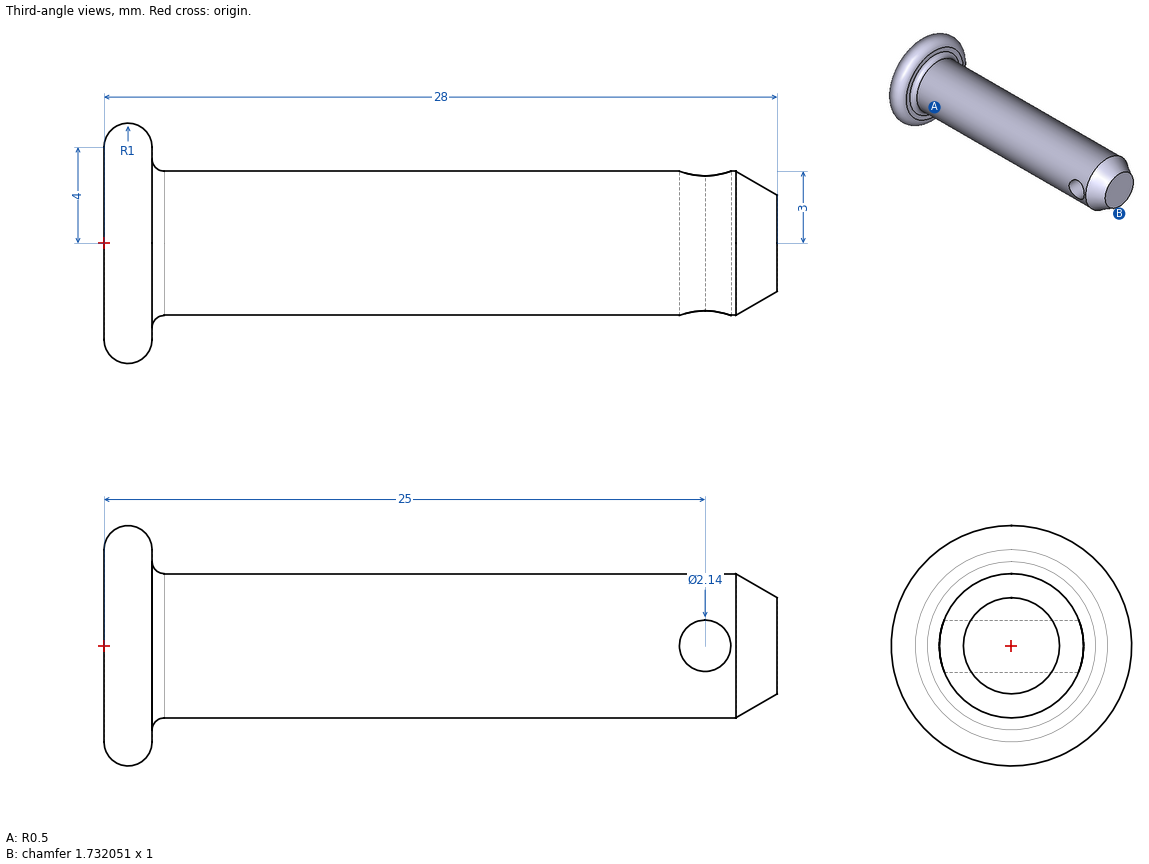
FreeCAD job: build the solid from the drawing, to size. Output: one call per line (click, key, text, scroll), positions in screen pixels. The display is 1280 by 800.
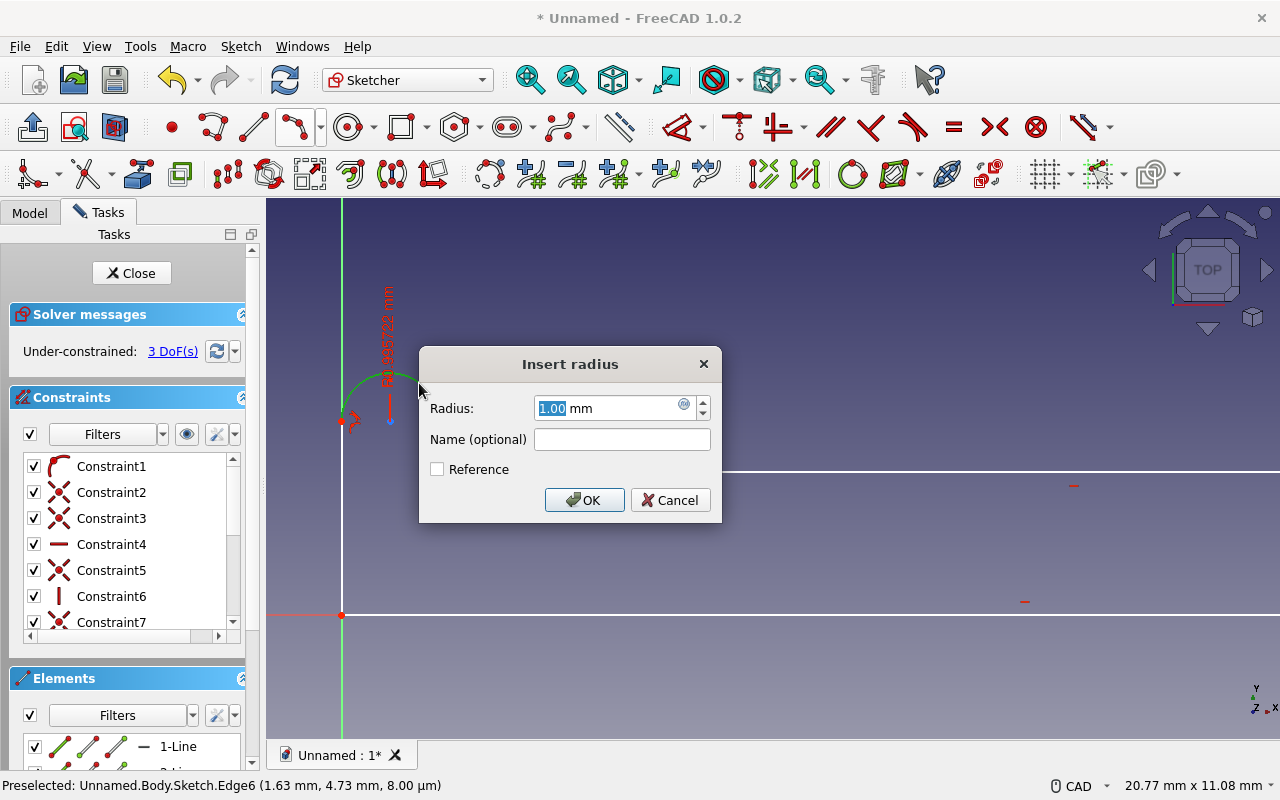
text(1)
key(Return)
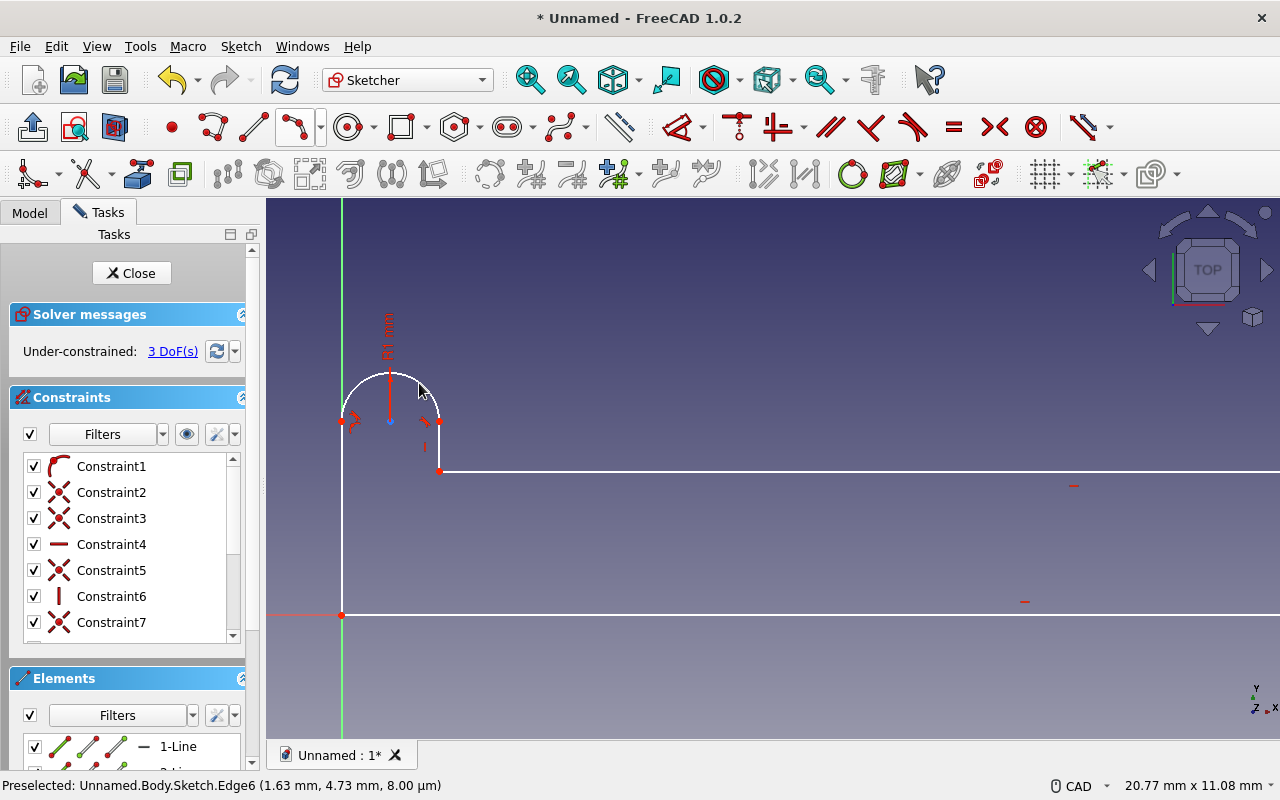
click(342, 480)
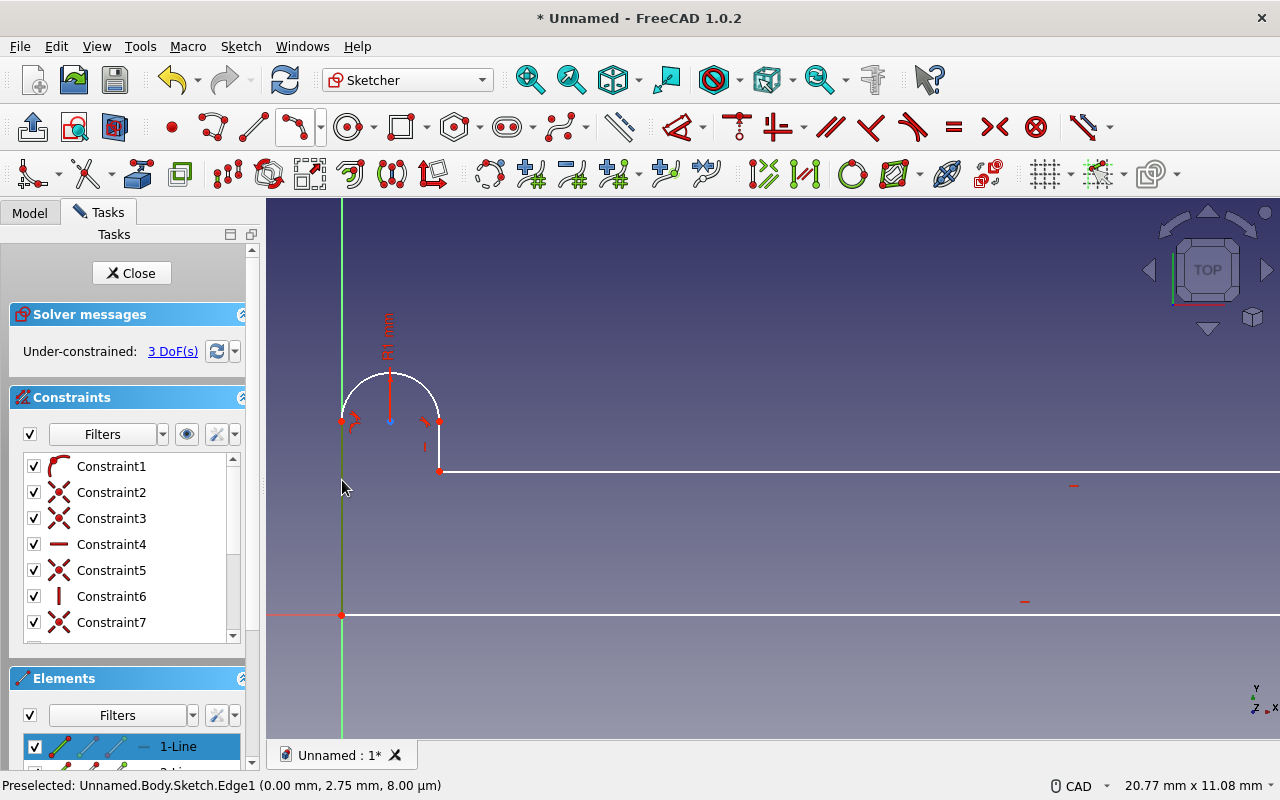
key(i)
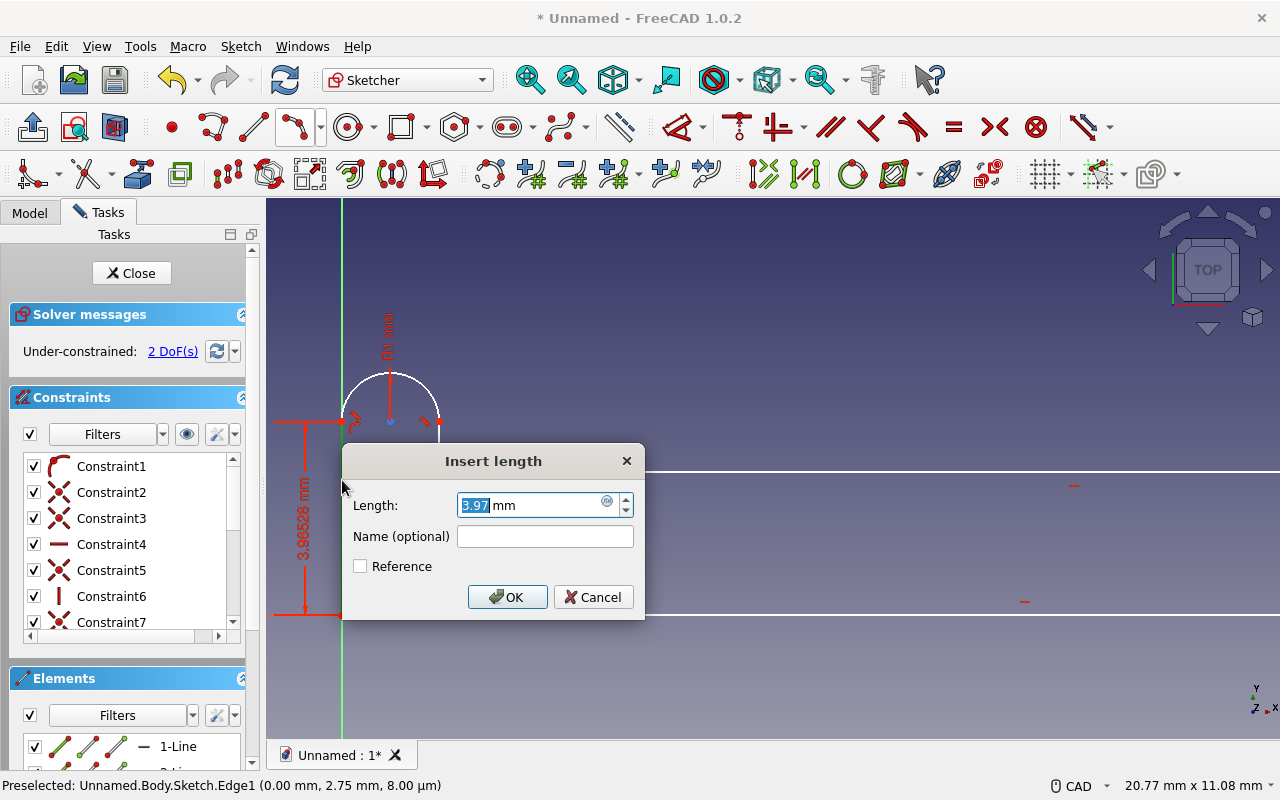
text(4)
key(Return)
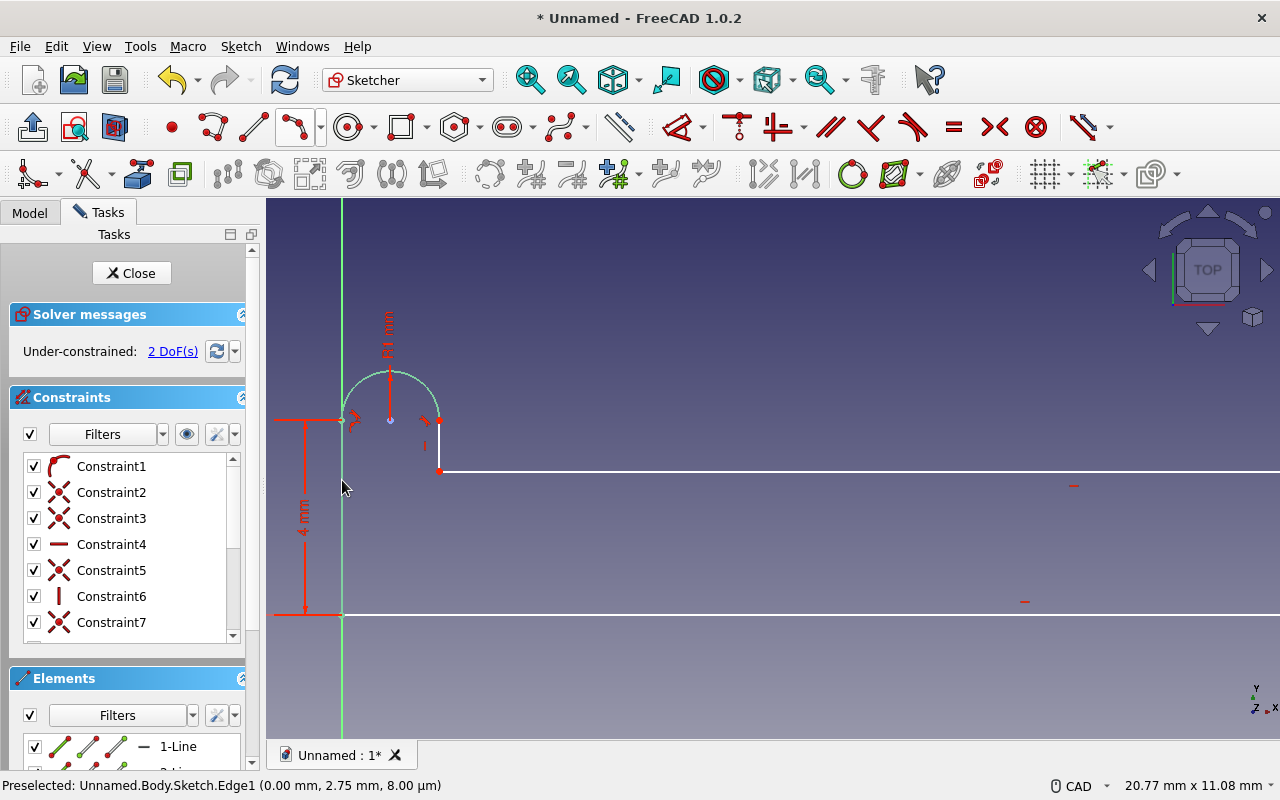
scroll(443, 448, down, 4)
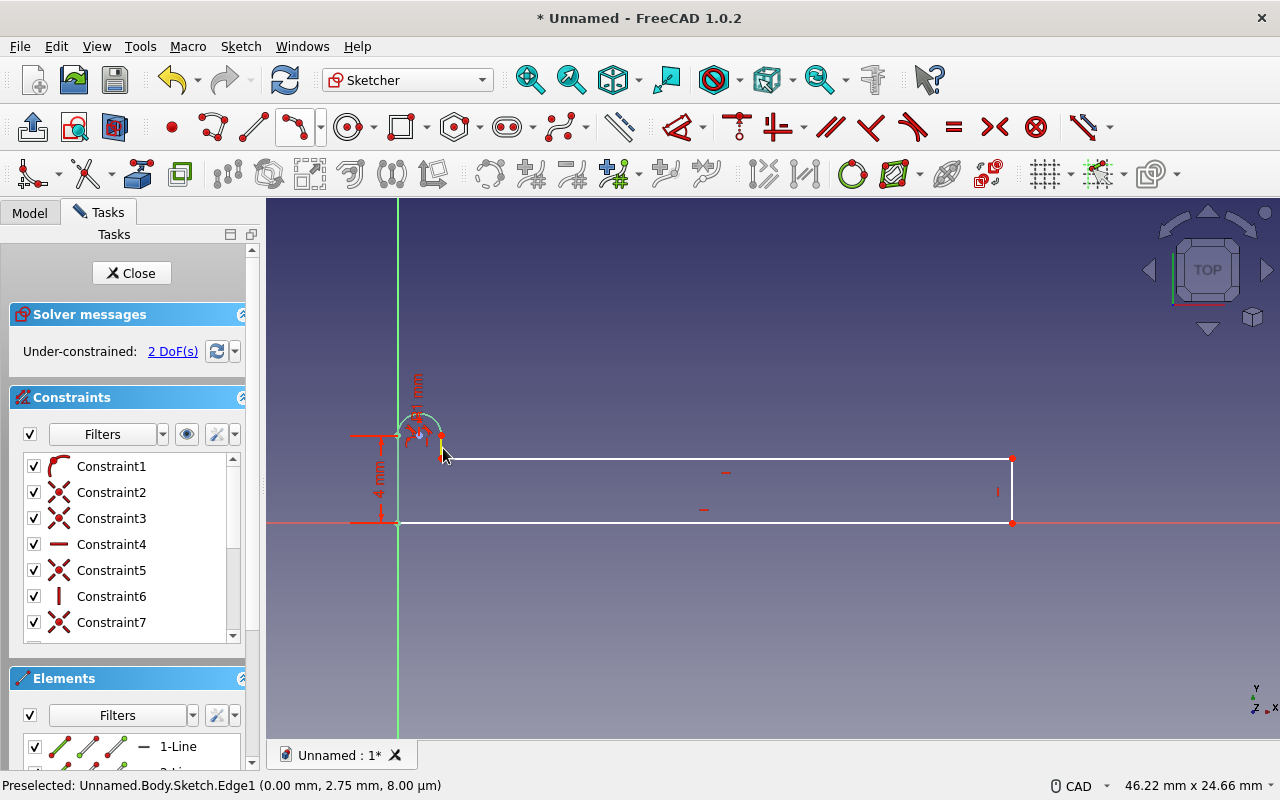
click(1012, 504)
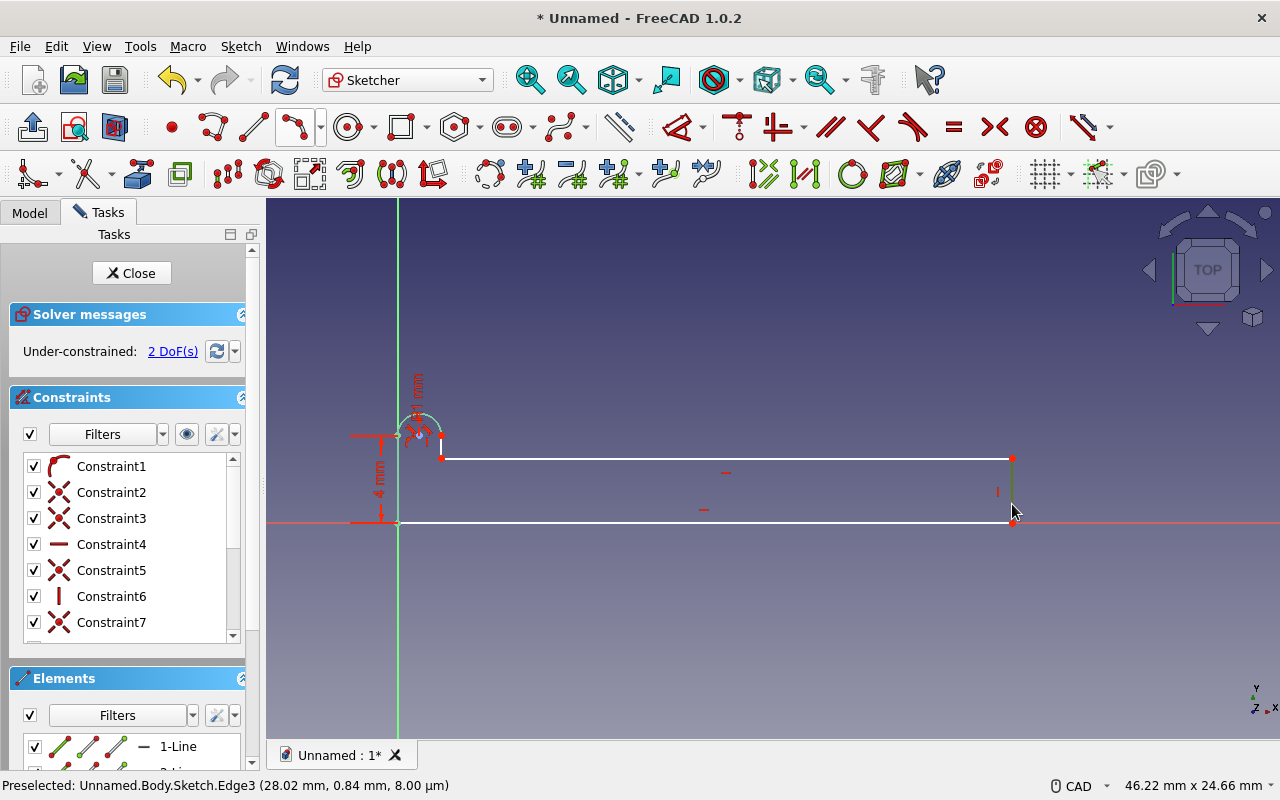
key(i)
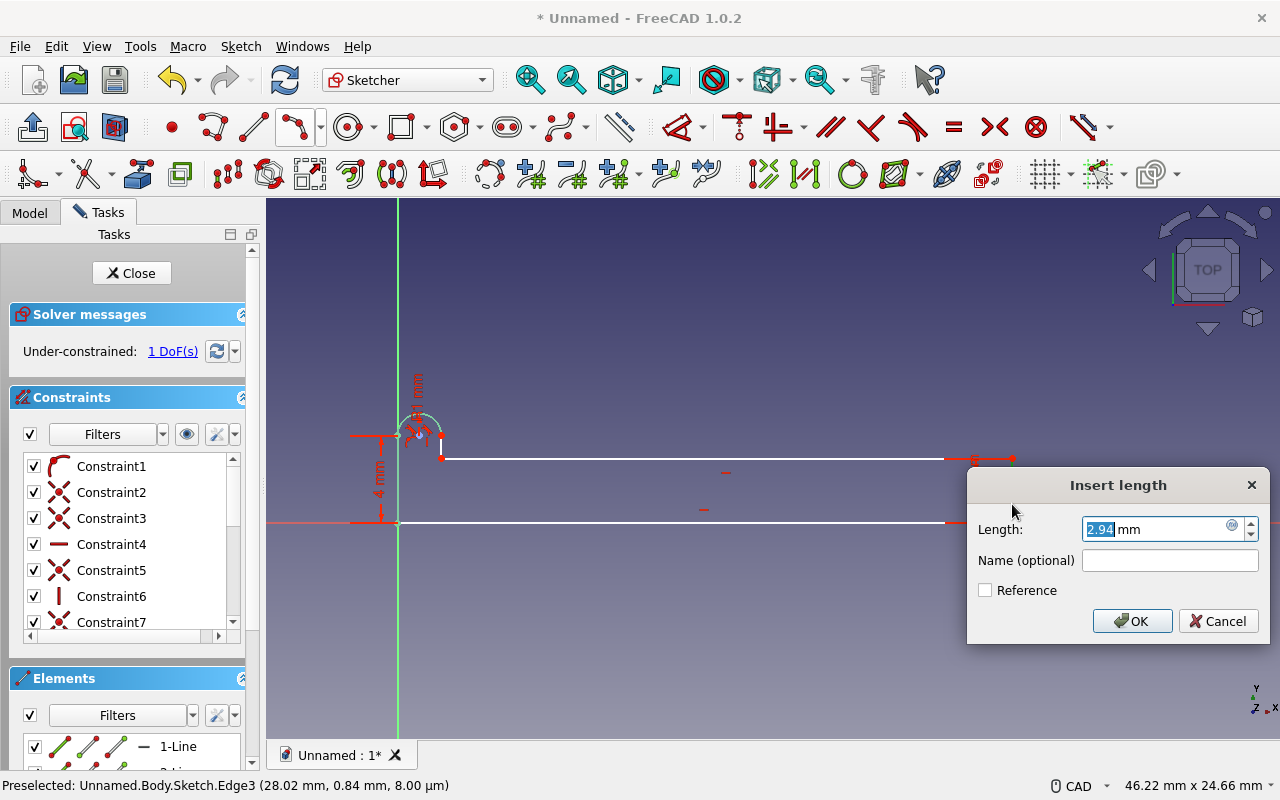
text(3)
key(Return)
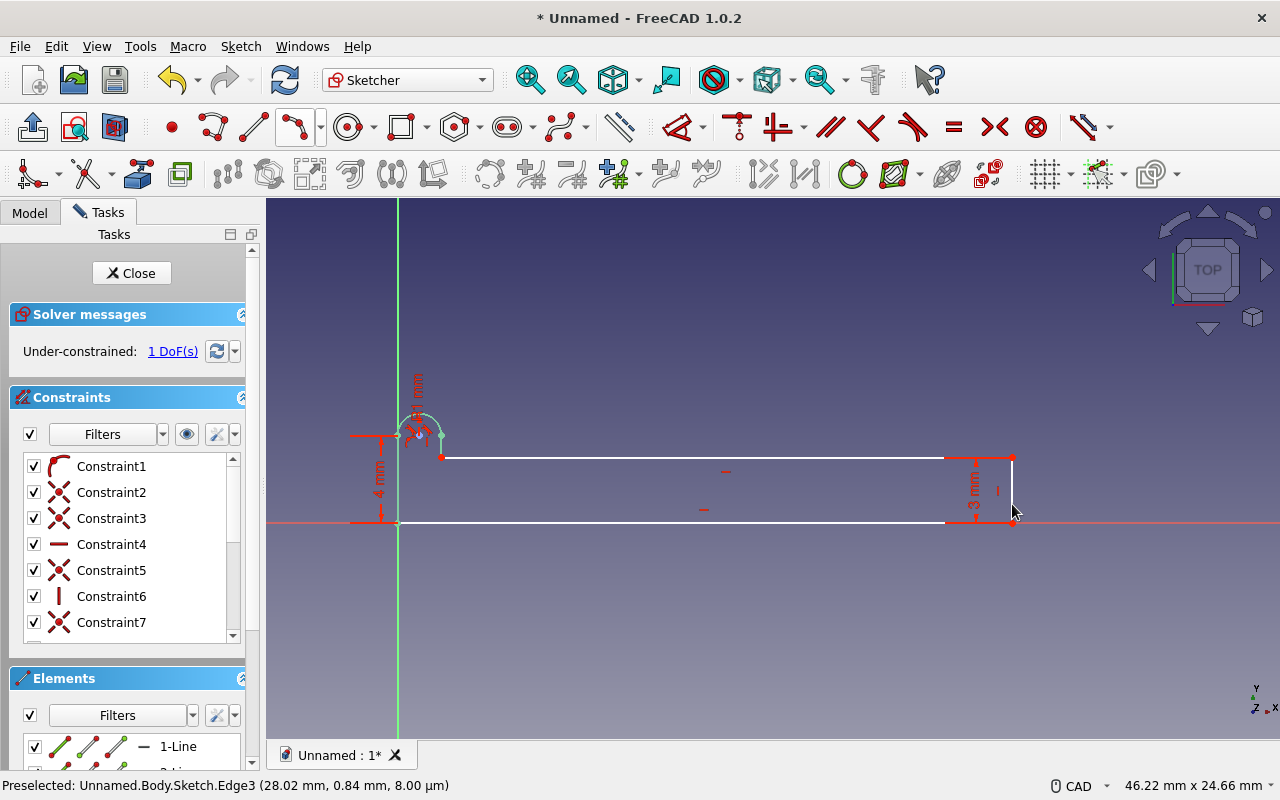
click(582, 523)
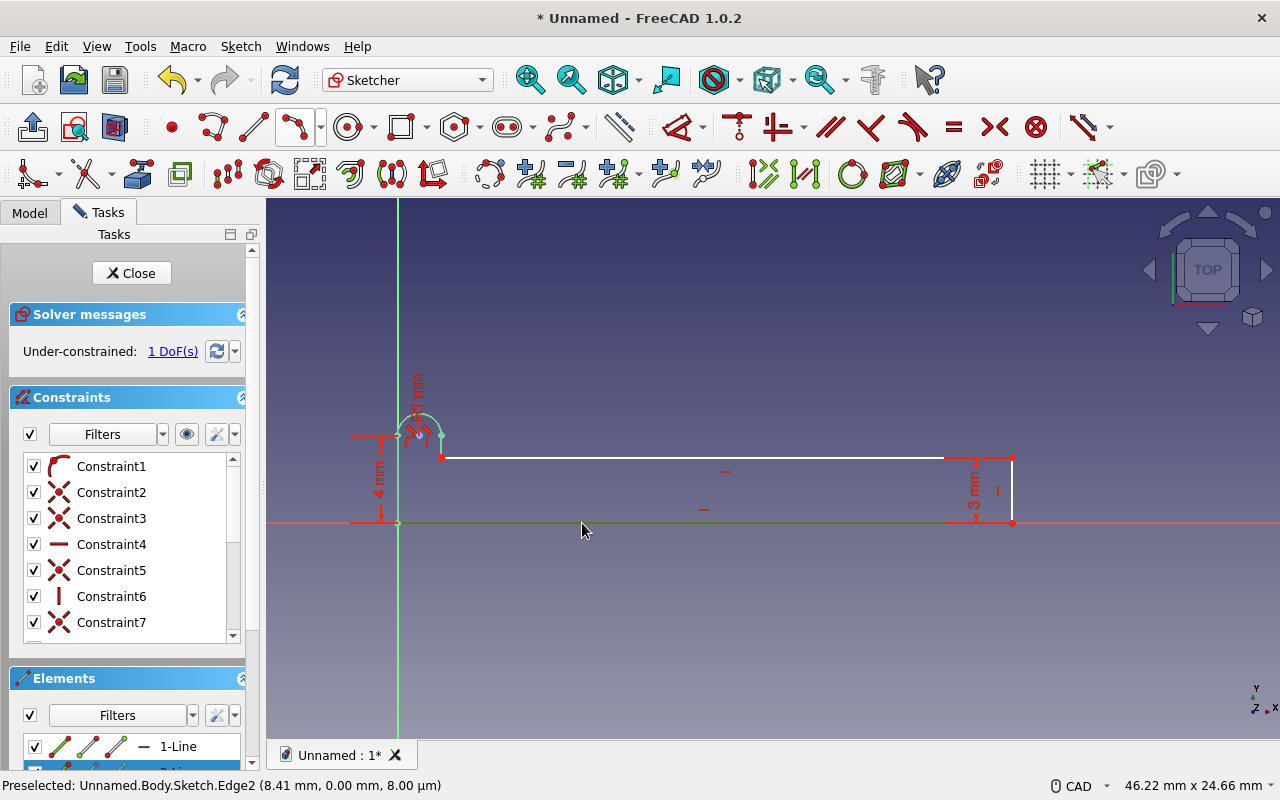
click(702, 128)